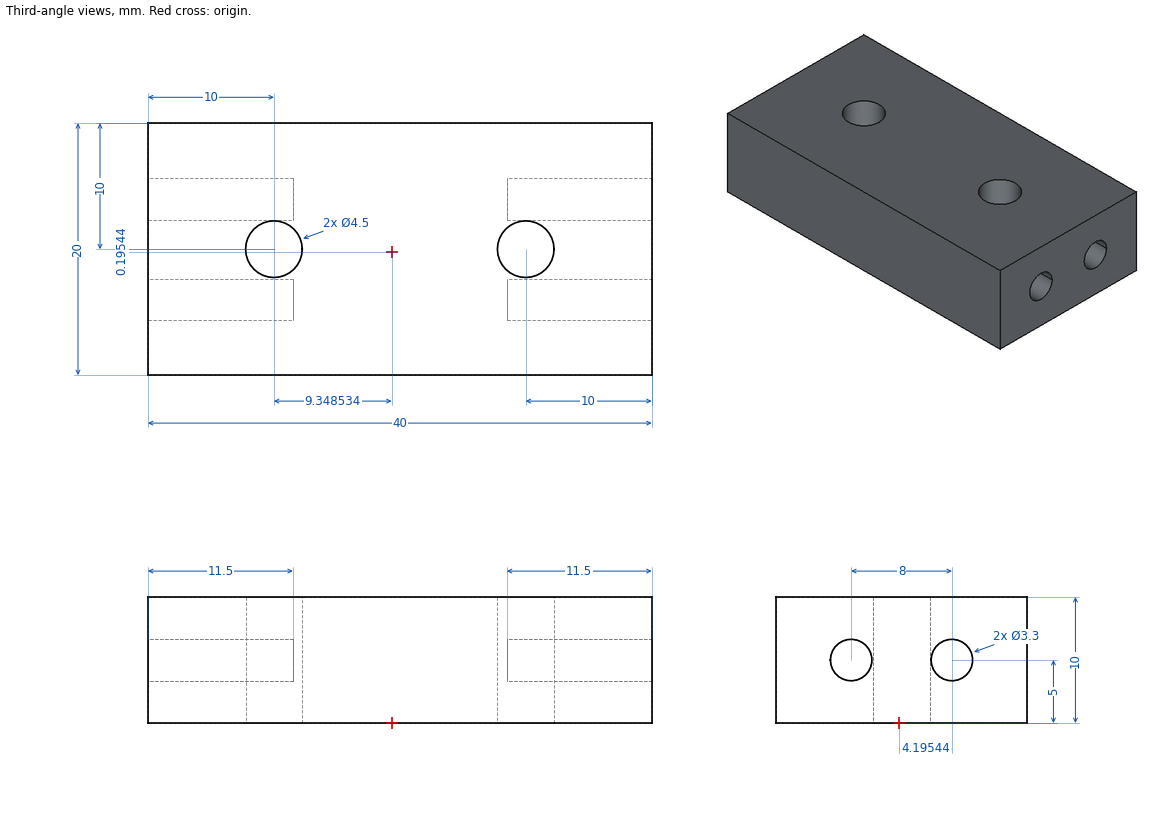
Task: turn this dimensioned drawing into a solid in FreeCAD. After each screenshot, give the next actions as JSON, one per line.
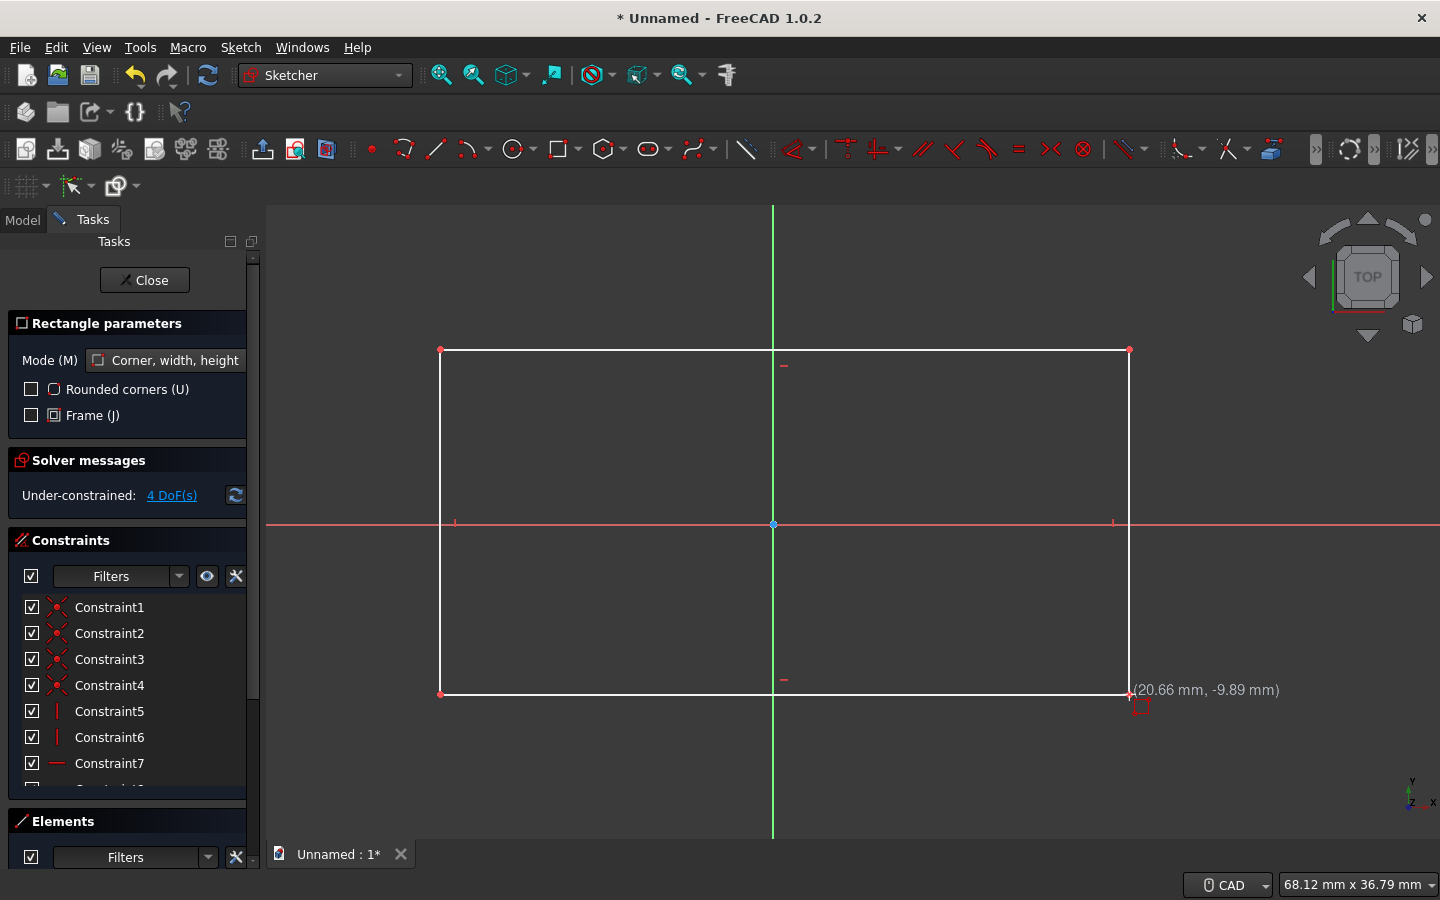
{"action": "left_click", "coordinate": [514, 150]}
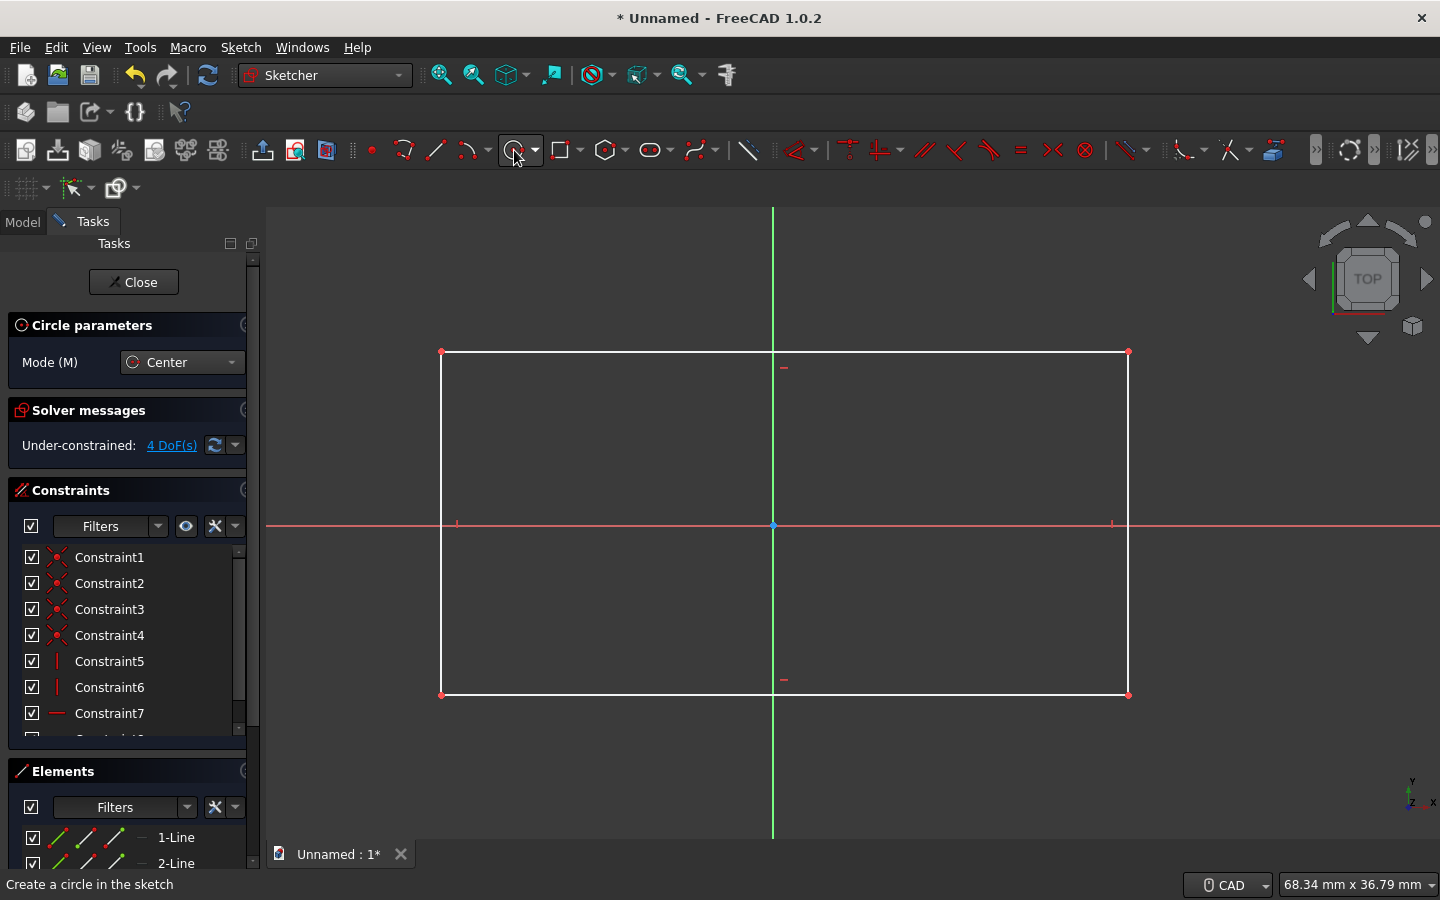
{"action": "scroll", "coordinate": [613, 522], "scroll_direction": "up", "scroll_amount": 8}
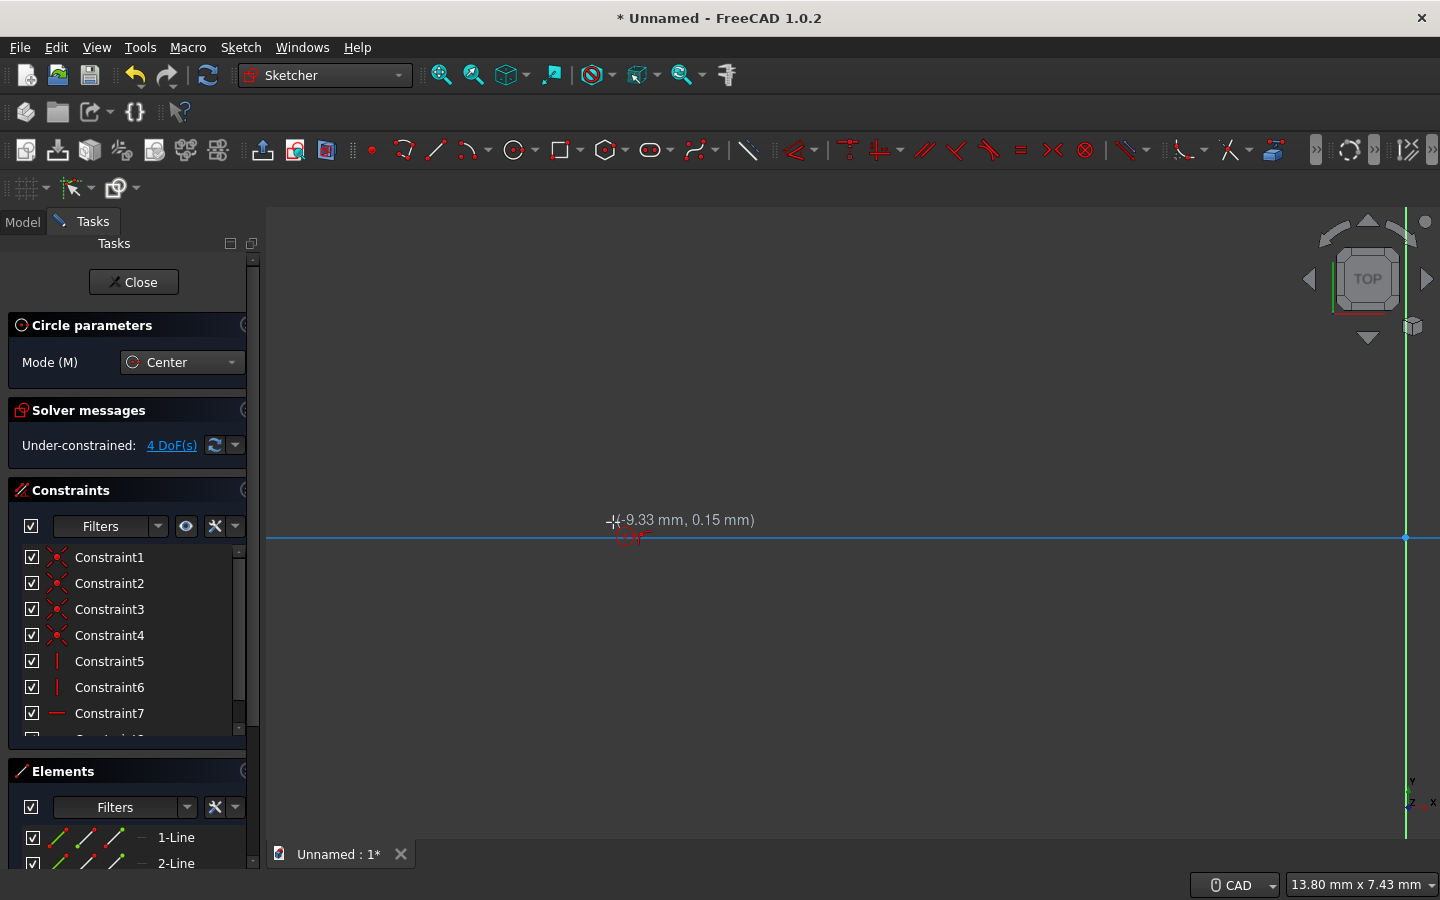
{"action": "left_click", "coordinate": [610, 521]}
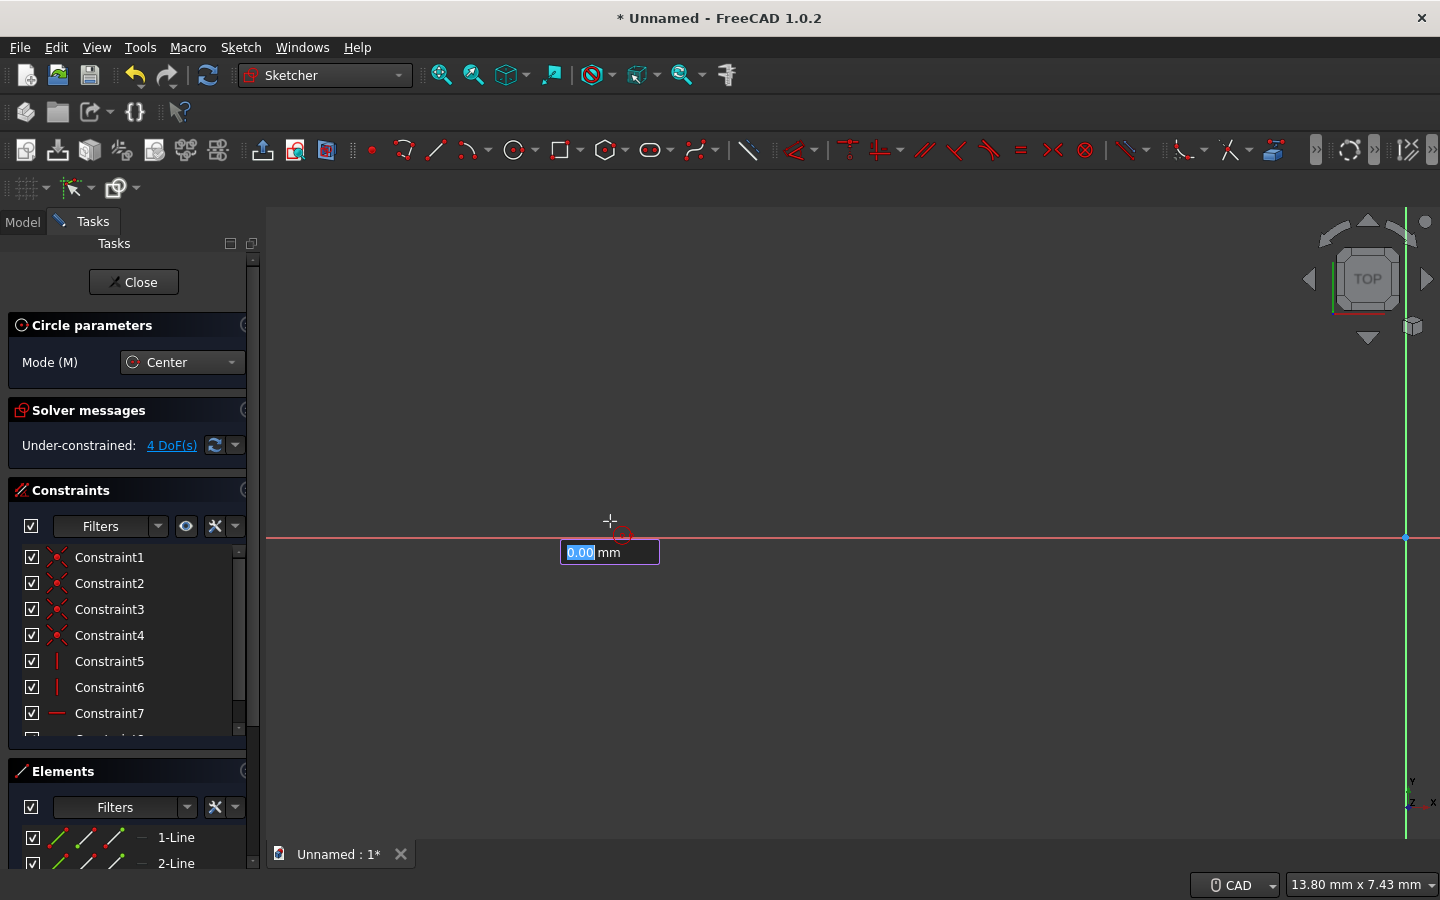
{"action": "scroll", "coordinate": [613, 523], "scroll_direction": "down", "scroll_amount": 8}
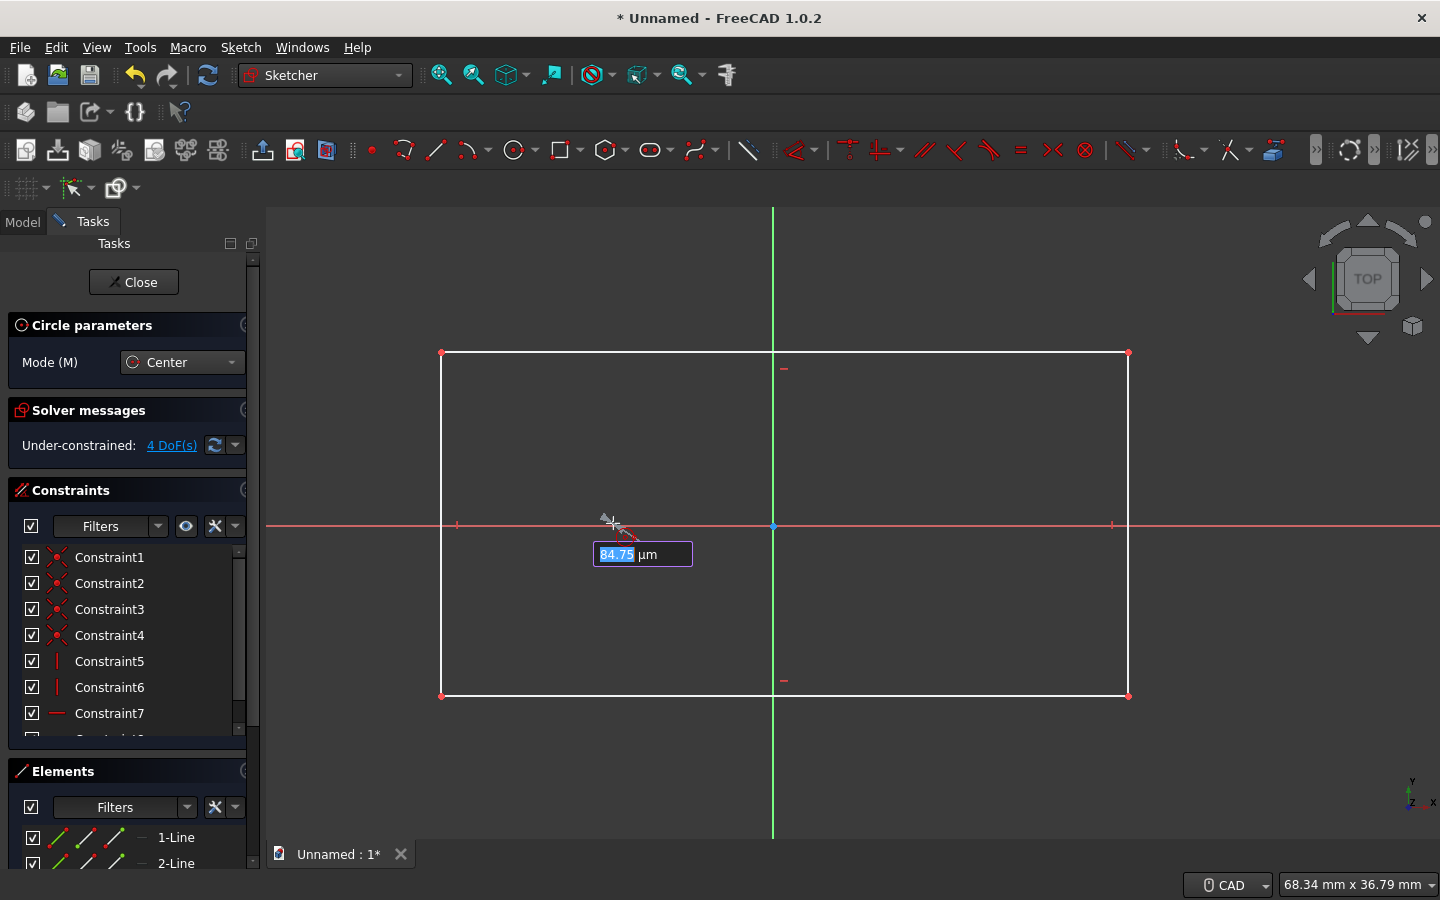
{"action": "left_click", "coordinate": [640, 496]}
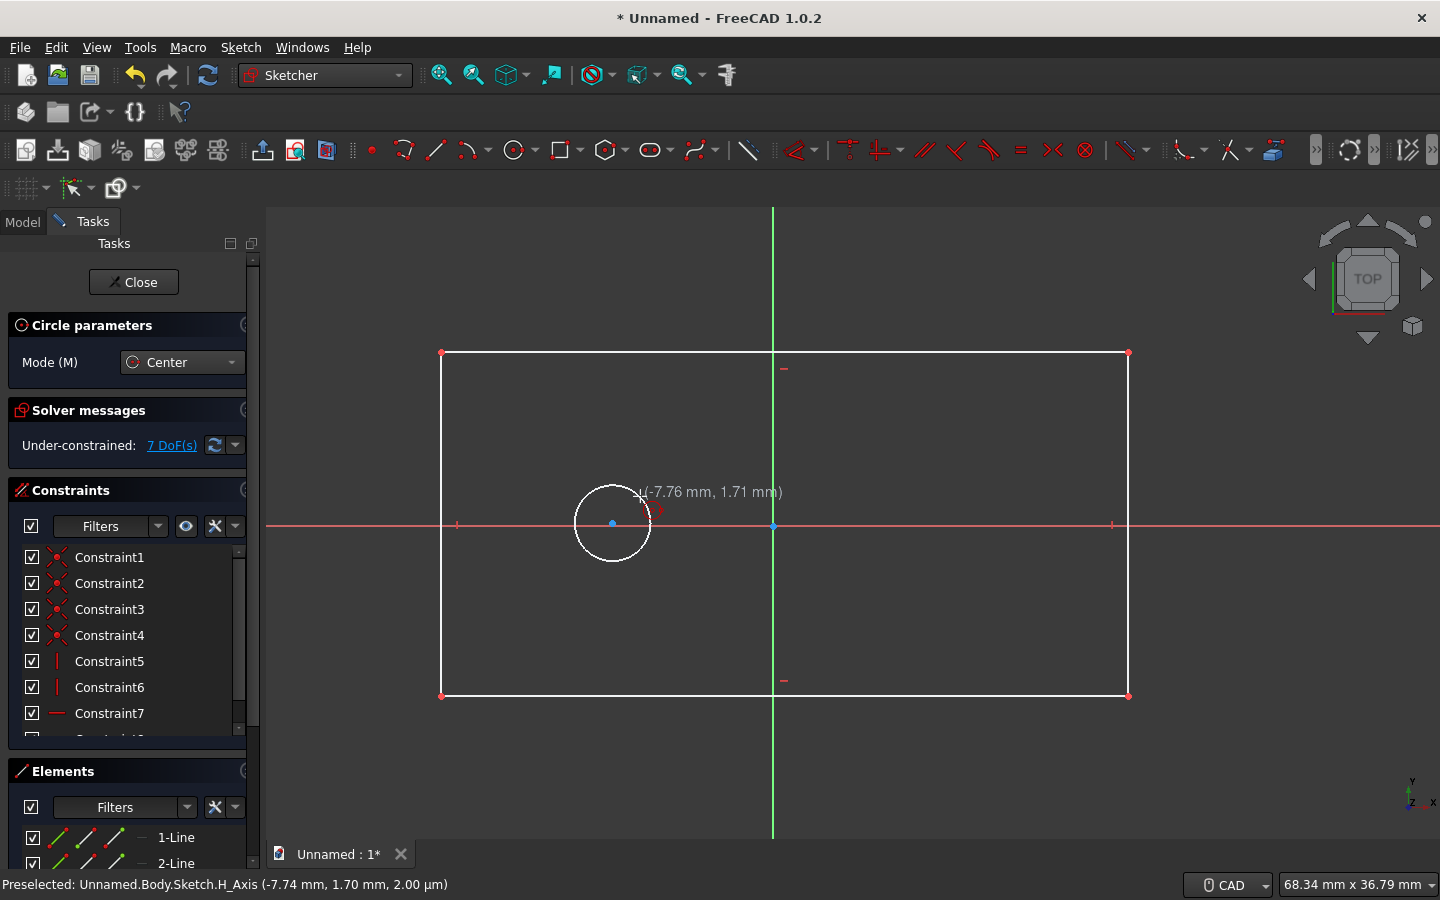
{"action": "scroll", "coordinate": [956, 523], "scroll_direction": "up", "scroll_amount": 8}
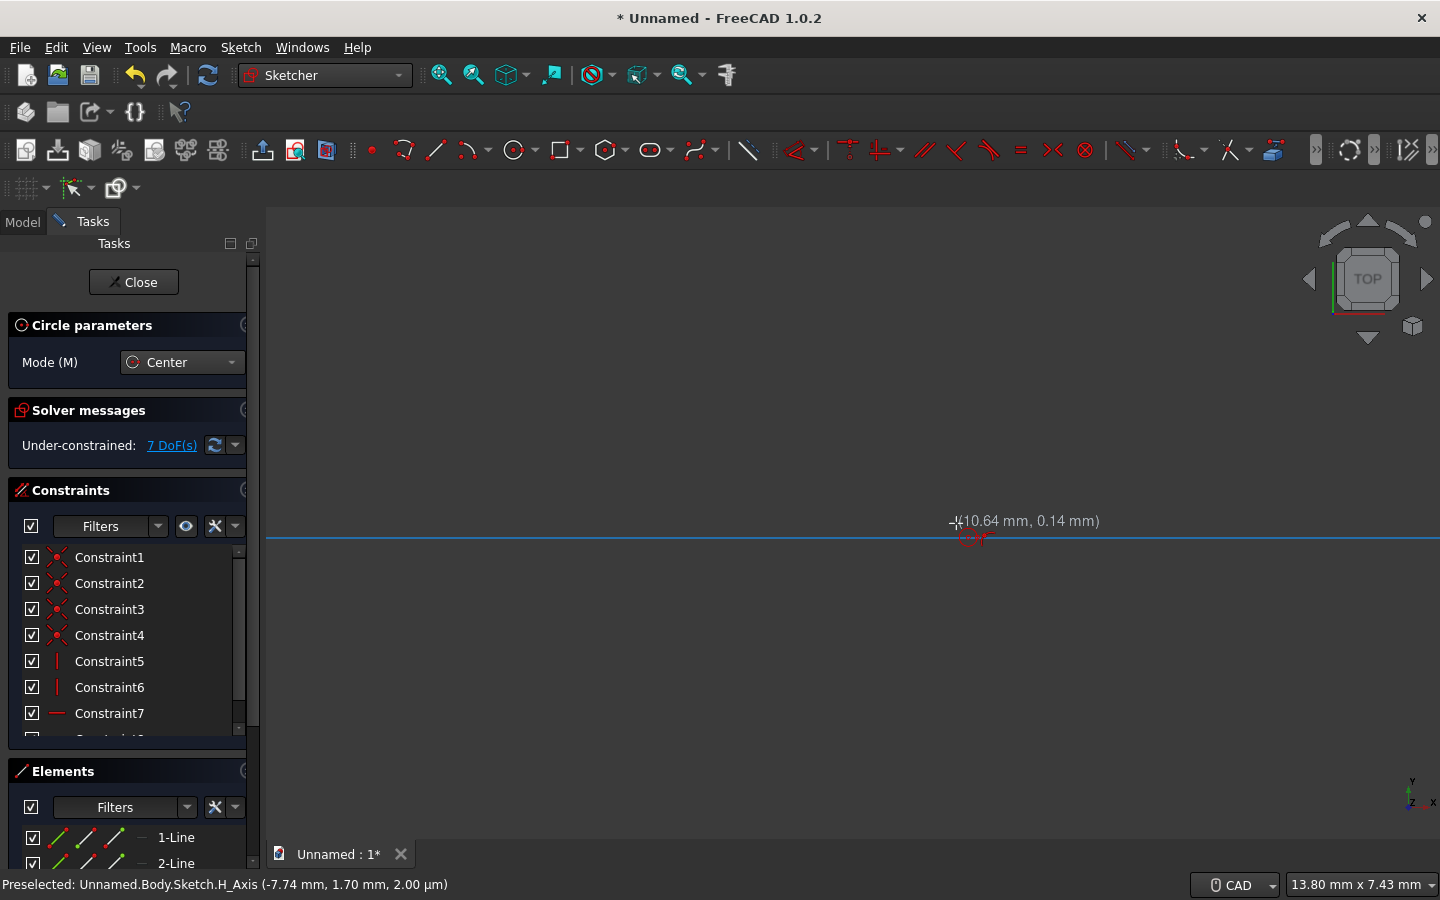
{"action": "left_click", "coordinate": [955, 521]}